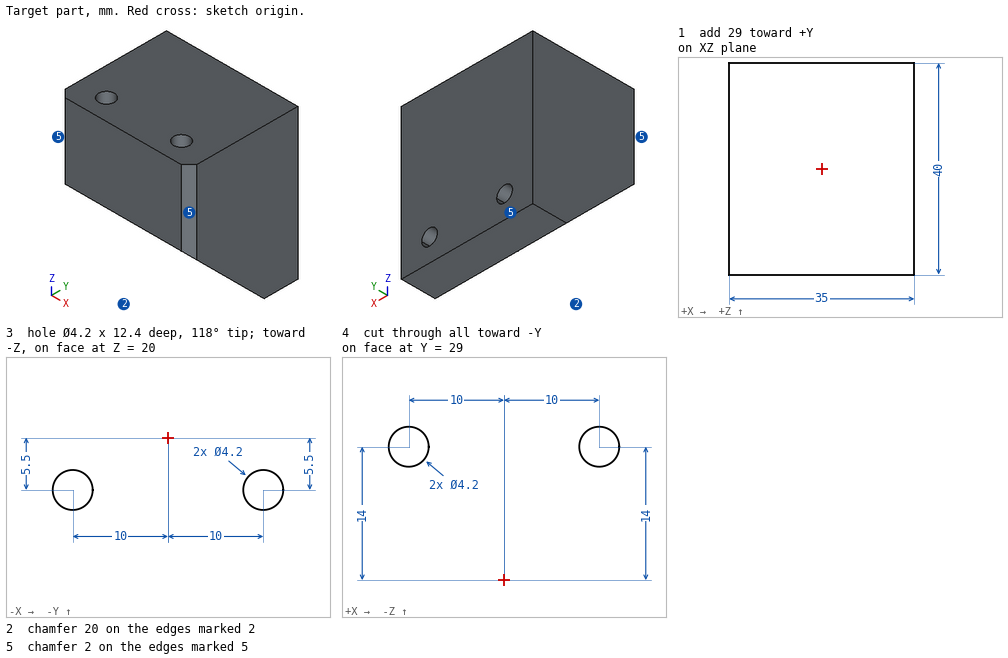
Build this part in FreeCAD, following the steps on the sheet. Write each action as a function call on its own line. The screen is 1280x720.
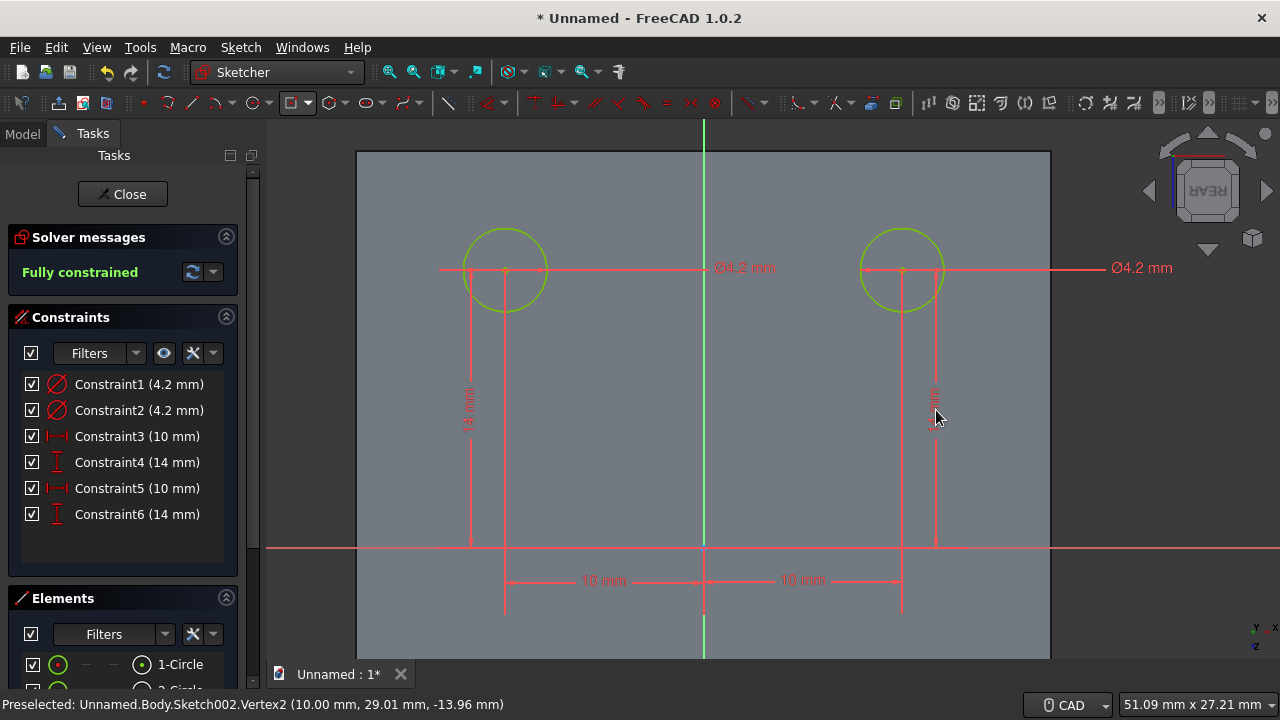
click(123, 194)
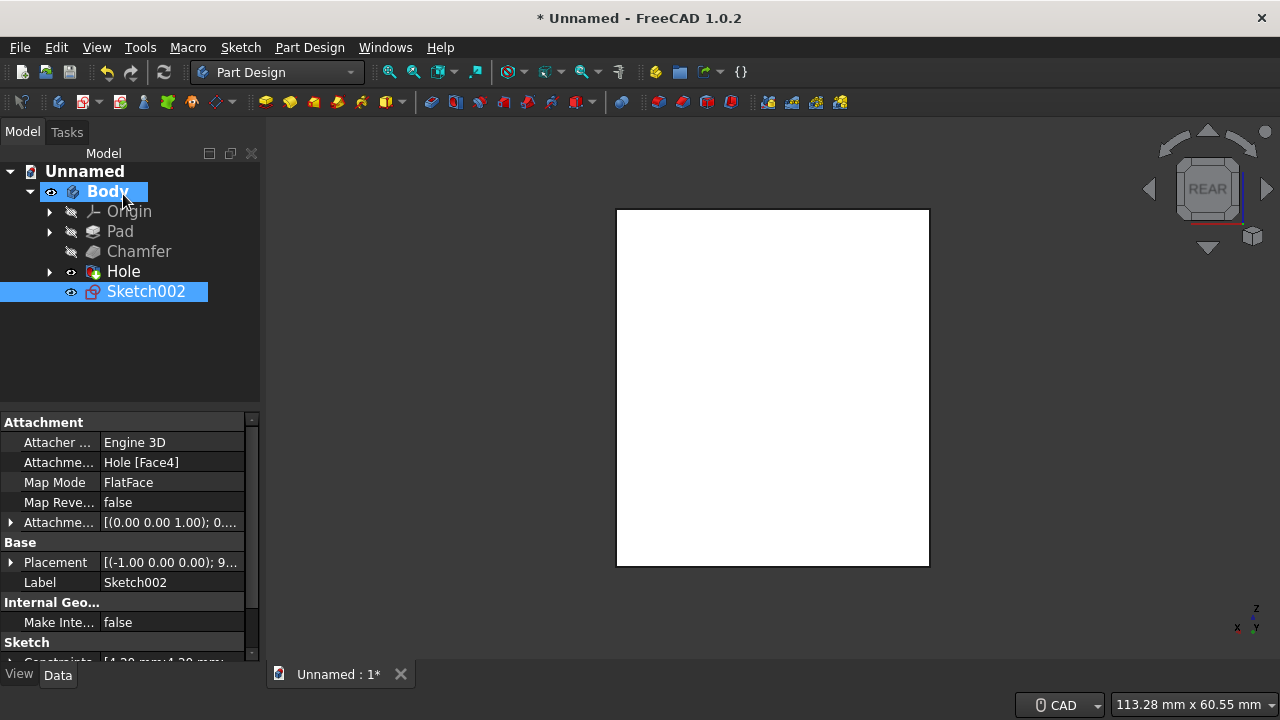
click(432, 102)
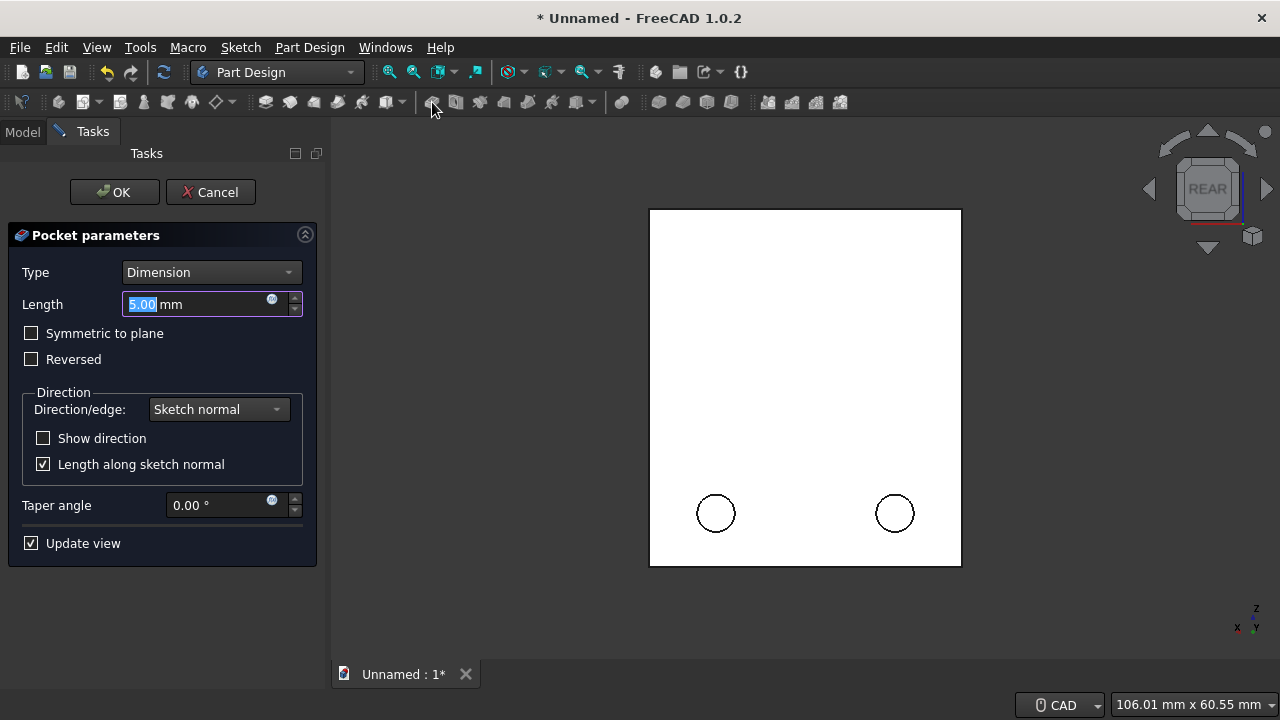
click(212, 272)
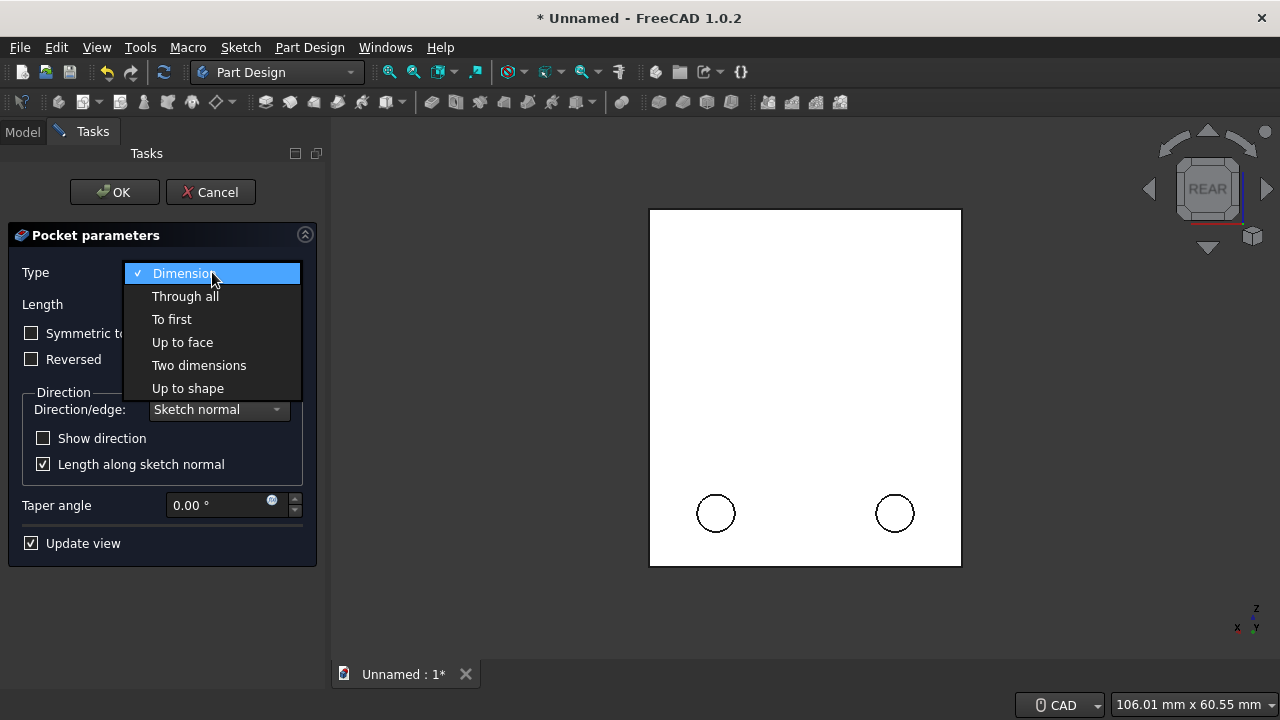
click(212, 296)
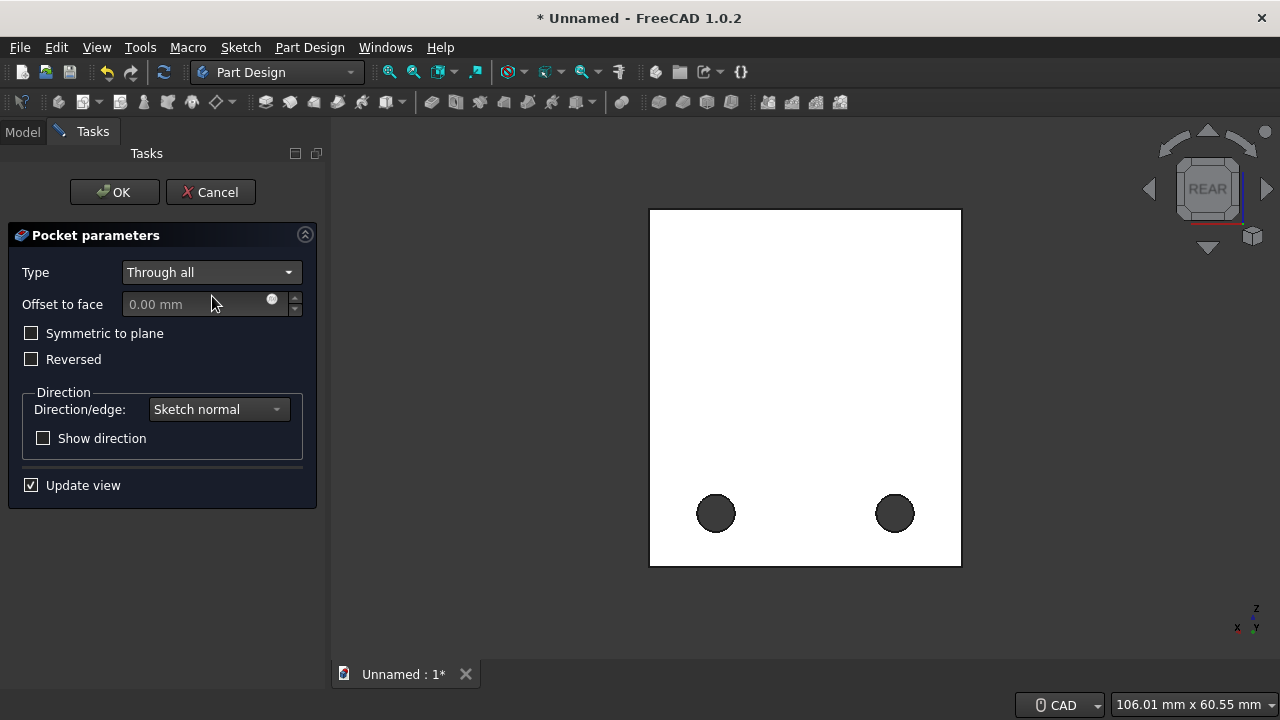
click(115, 192)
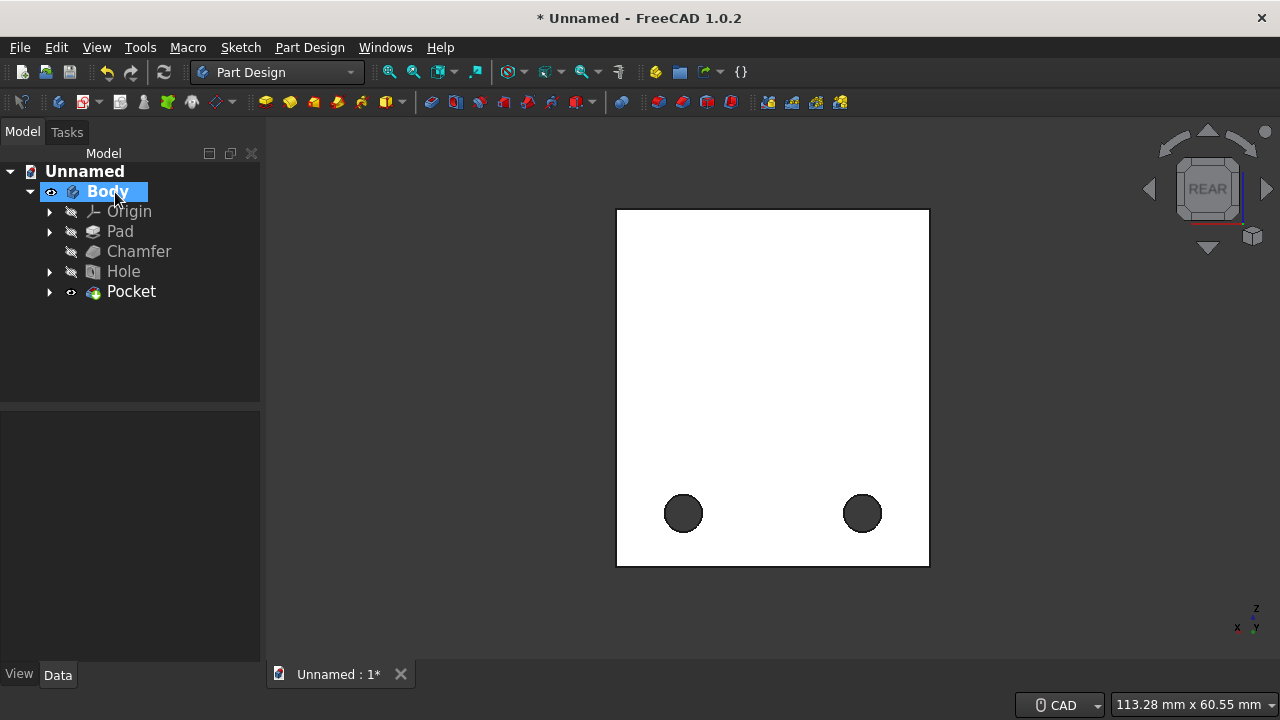
key(0)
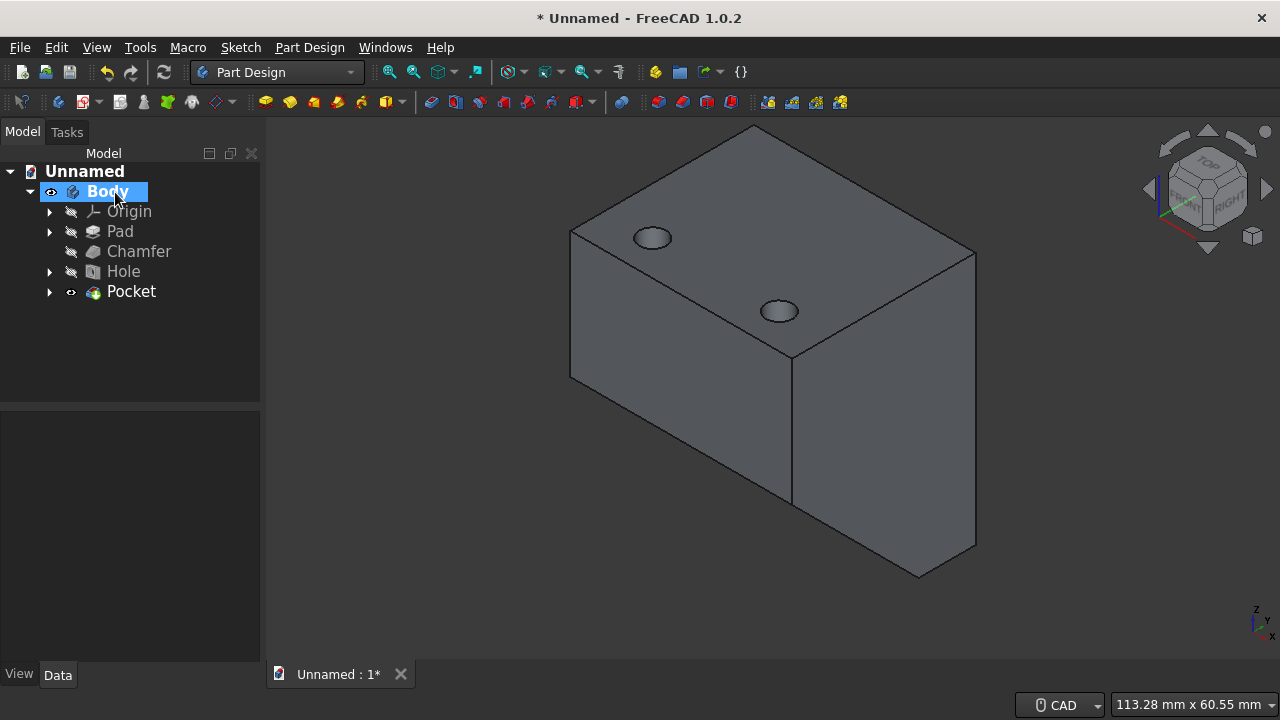
click(792, 431)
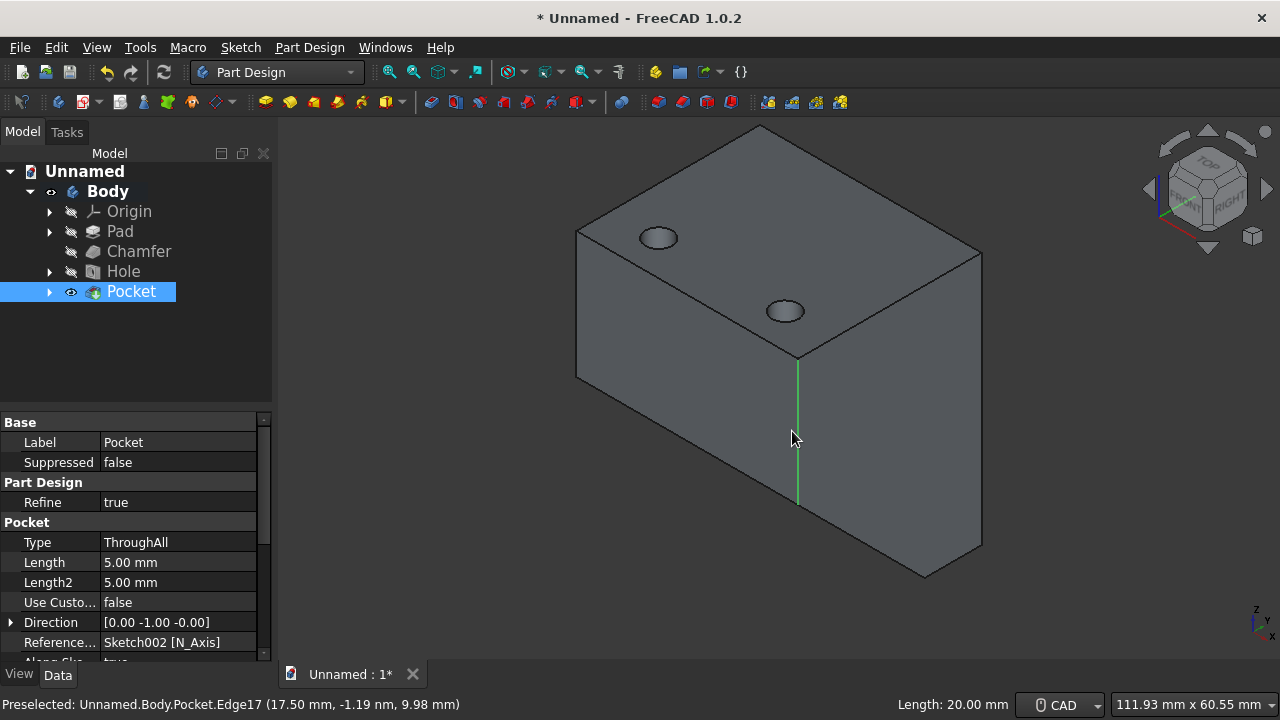
key(2)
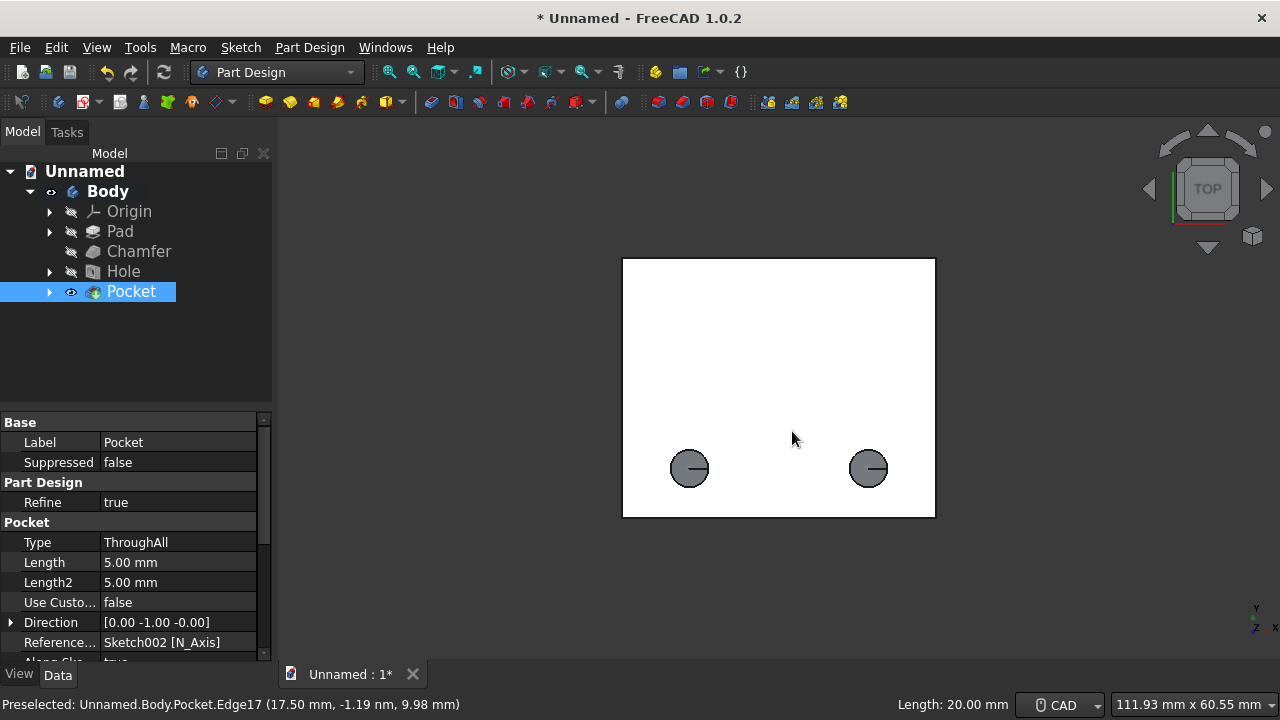
key(1)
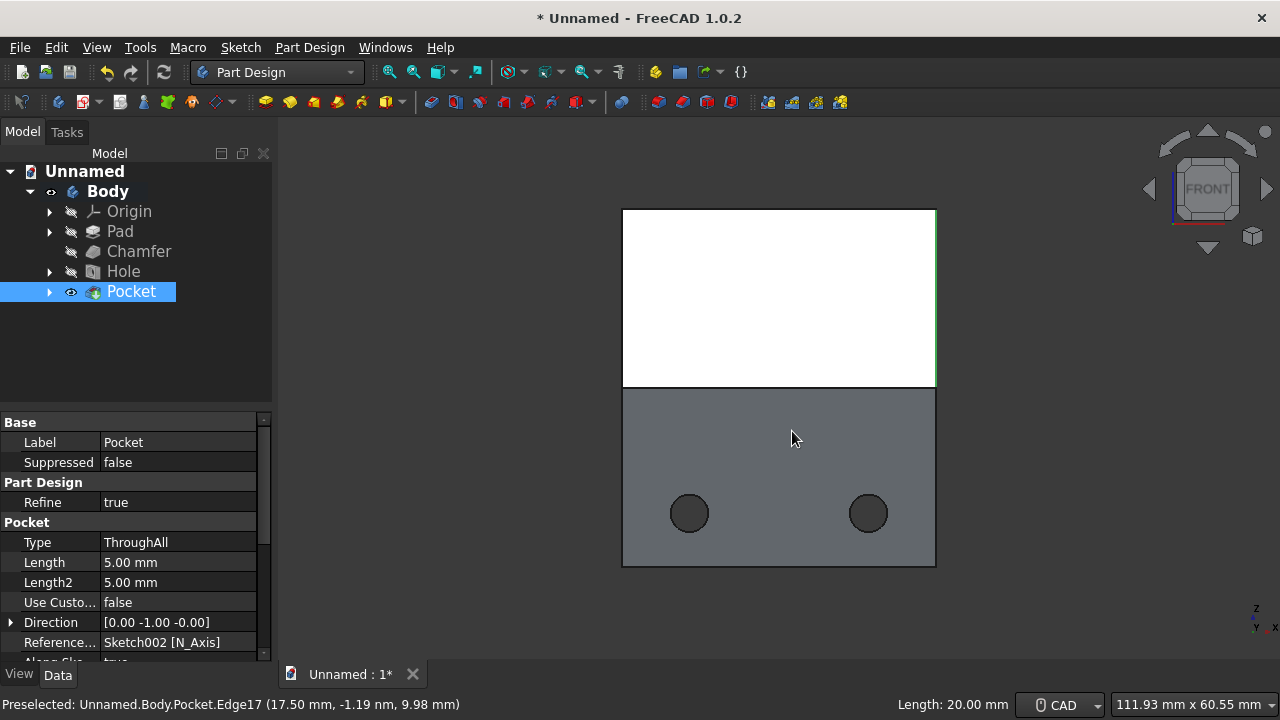
click(622, 297, ctrl)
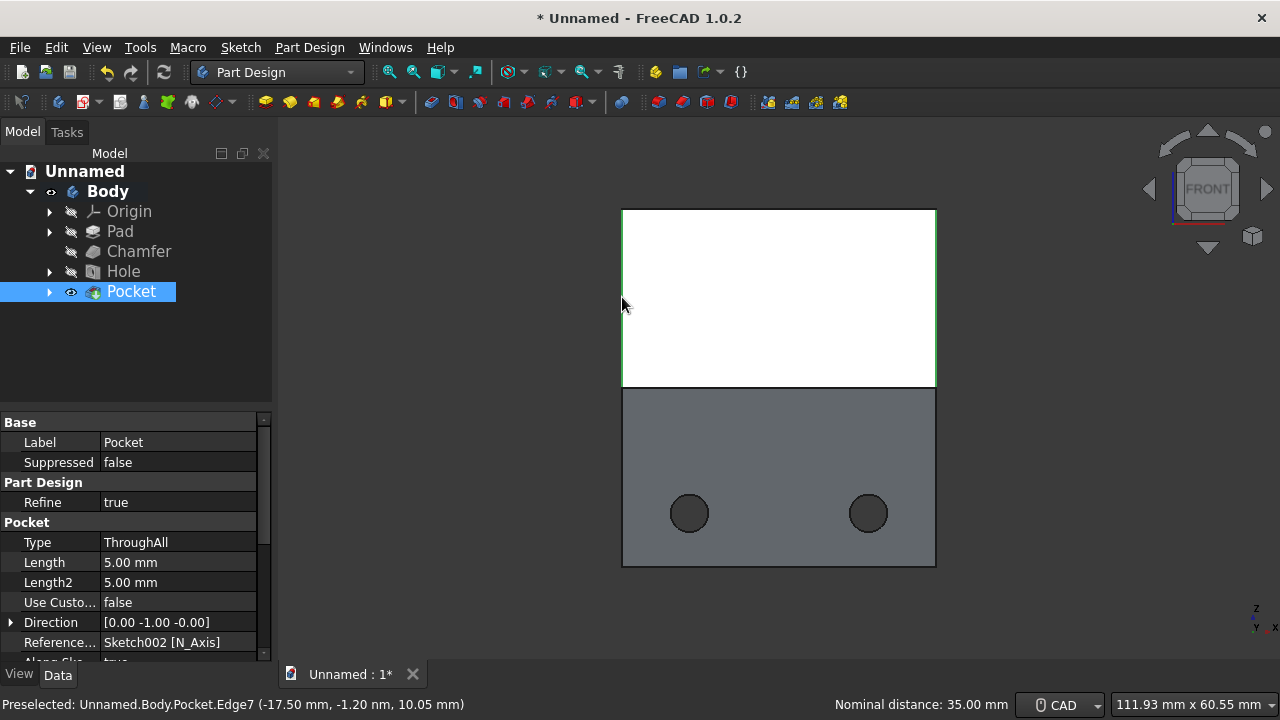
click(684, 102)